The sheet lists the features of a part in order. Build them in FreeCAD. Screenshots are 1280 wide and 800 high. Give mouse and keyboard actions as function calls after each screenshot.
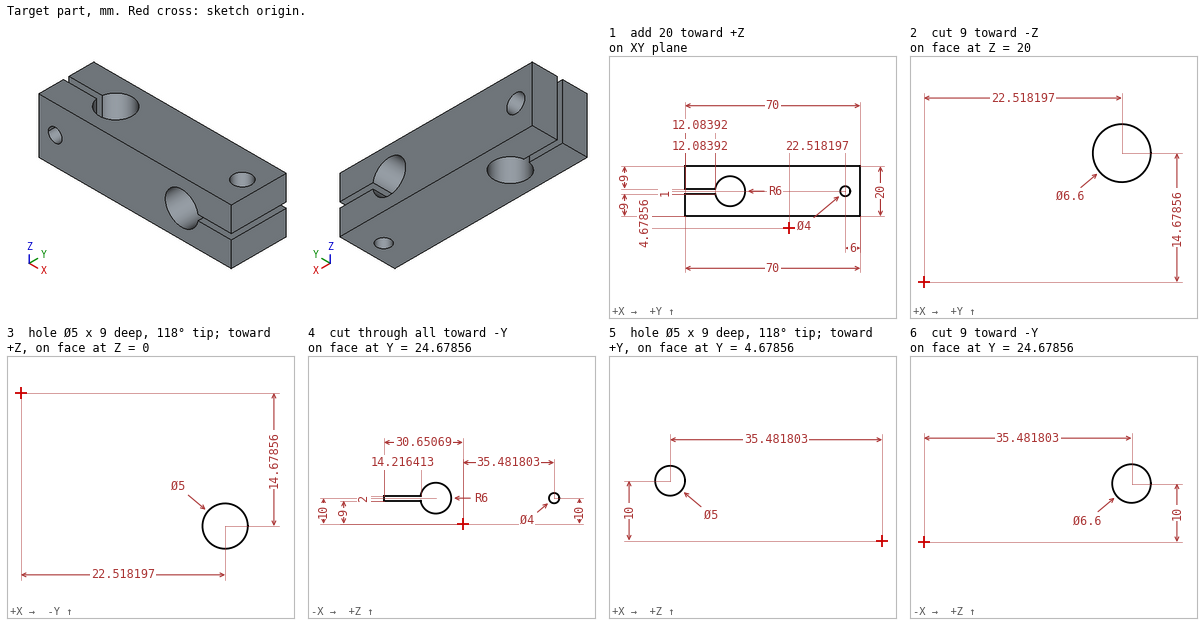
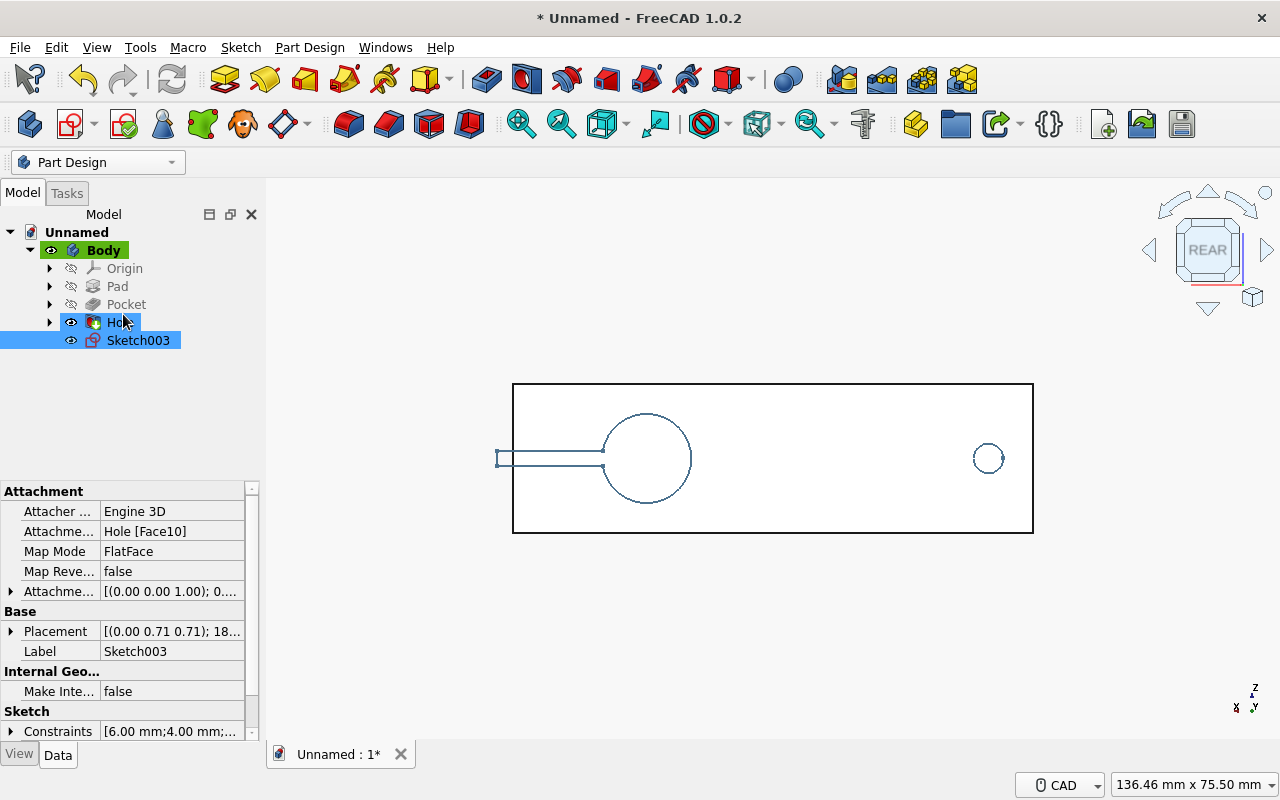
click(488, 80)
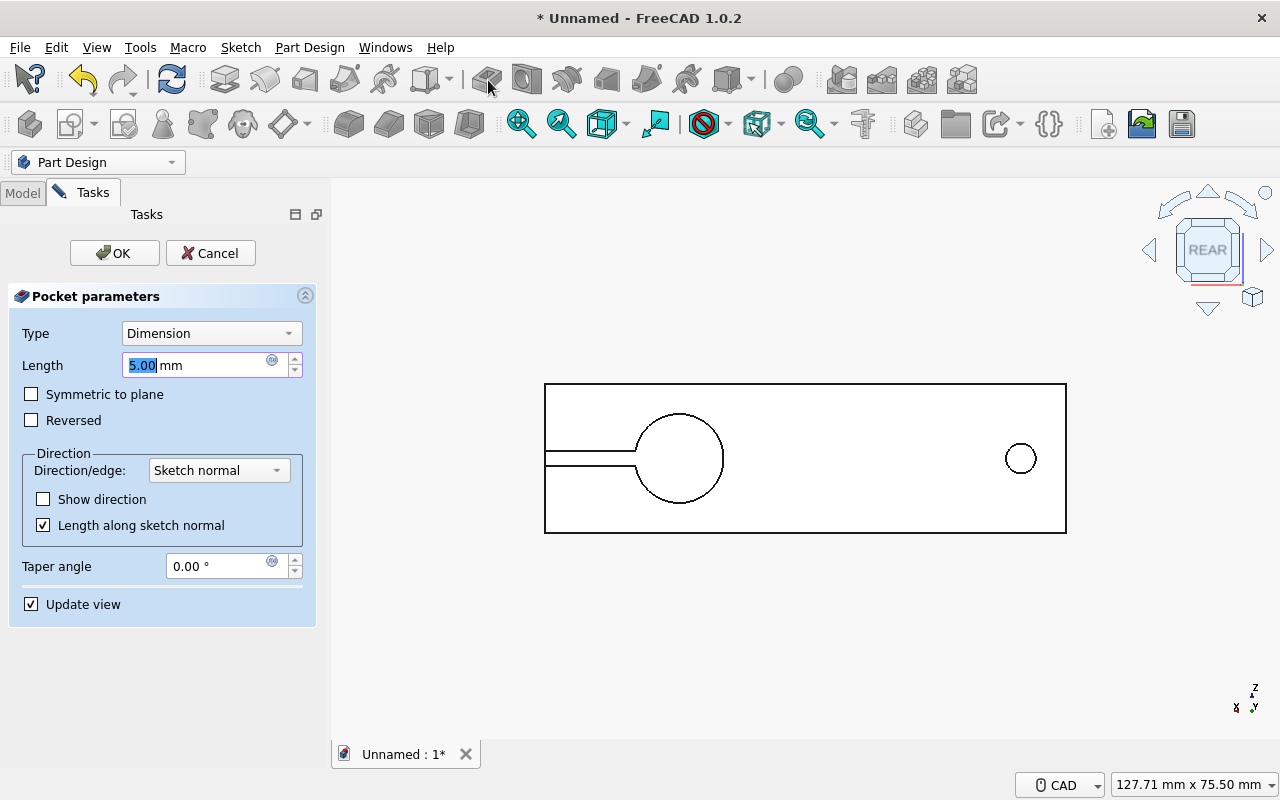
click(212, 334)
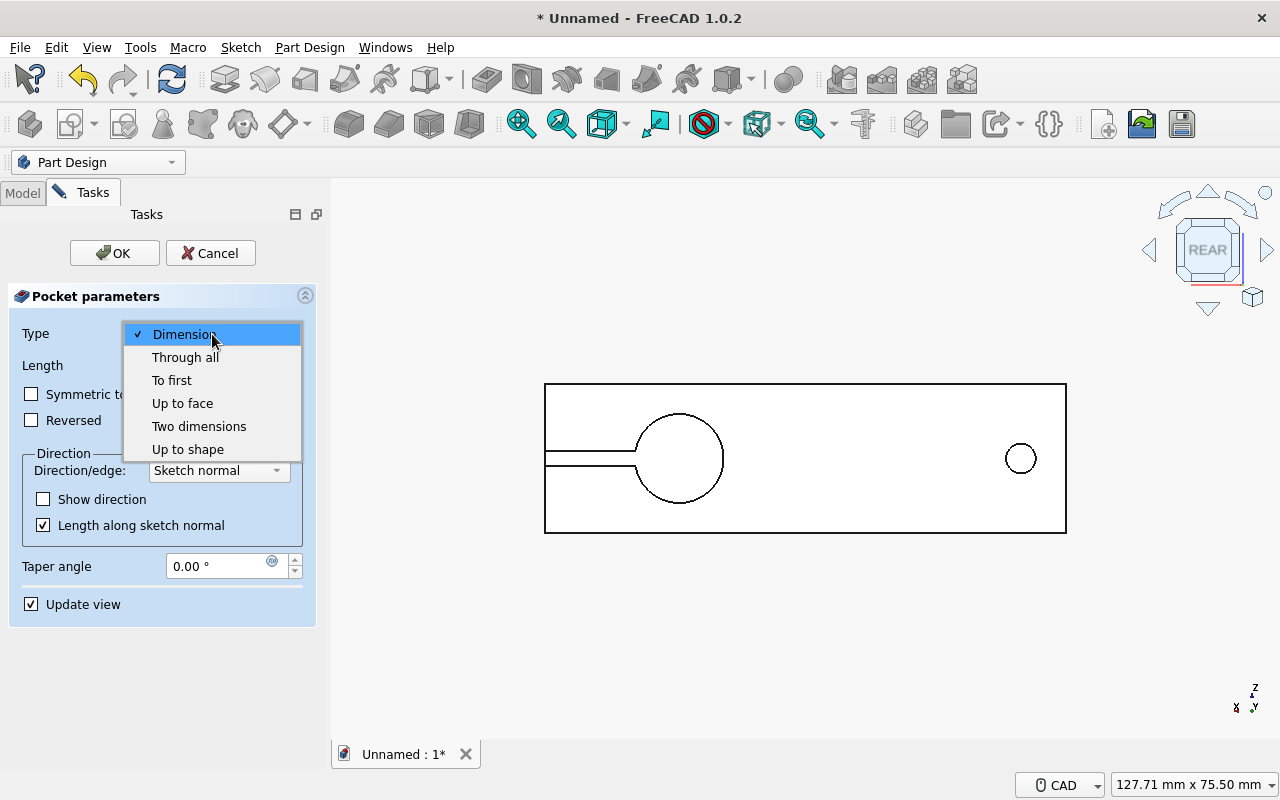
click(212, 358)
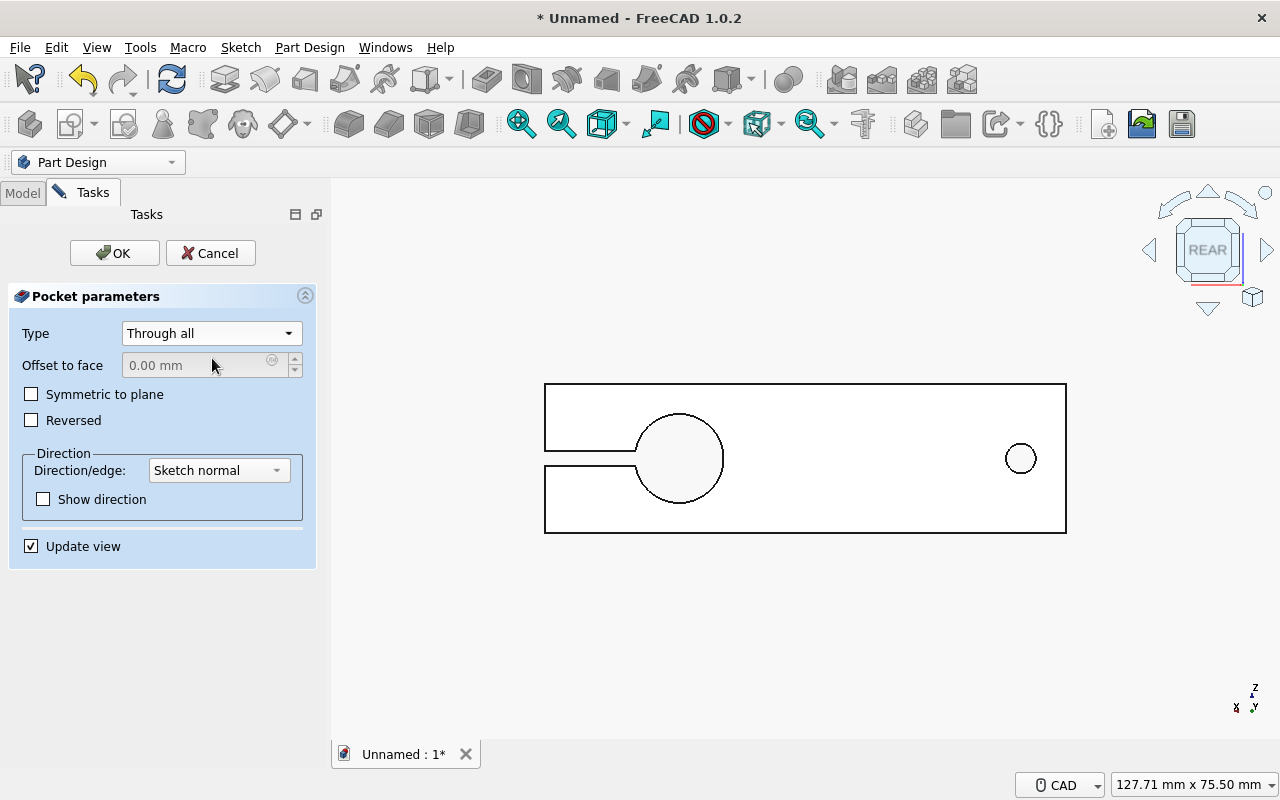
click(115, 253)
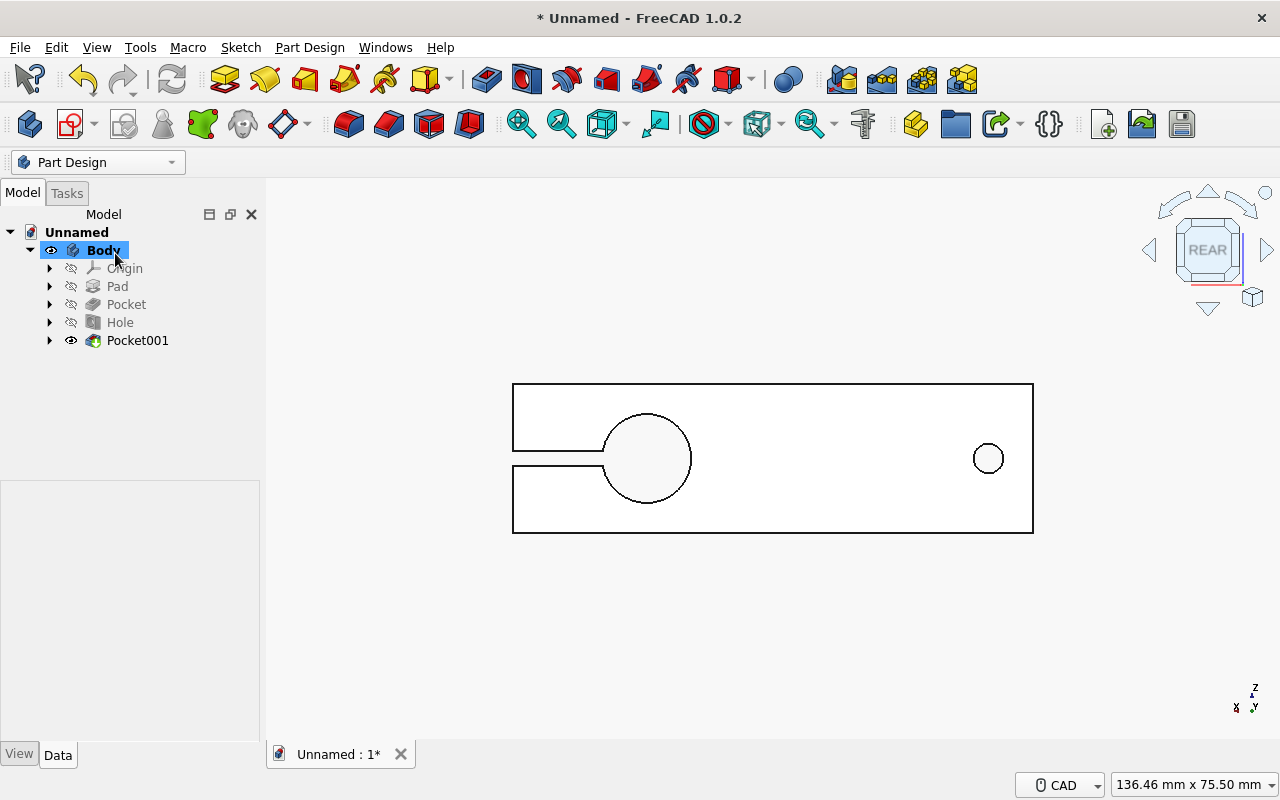
key(0)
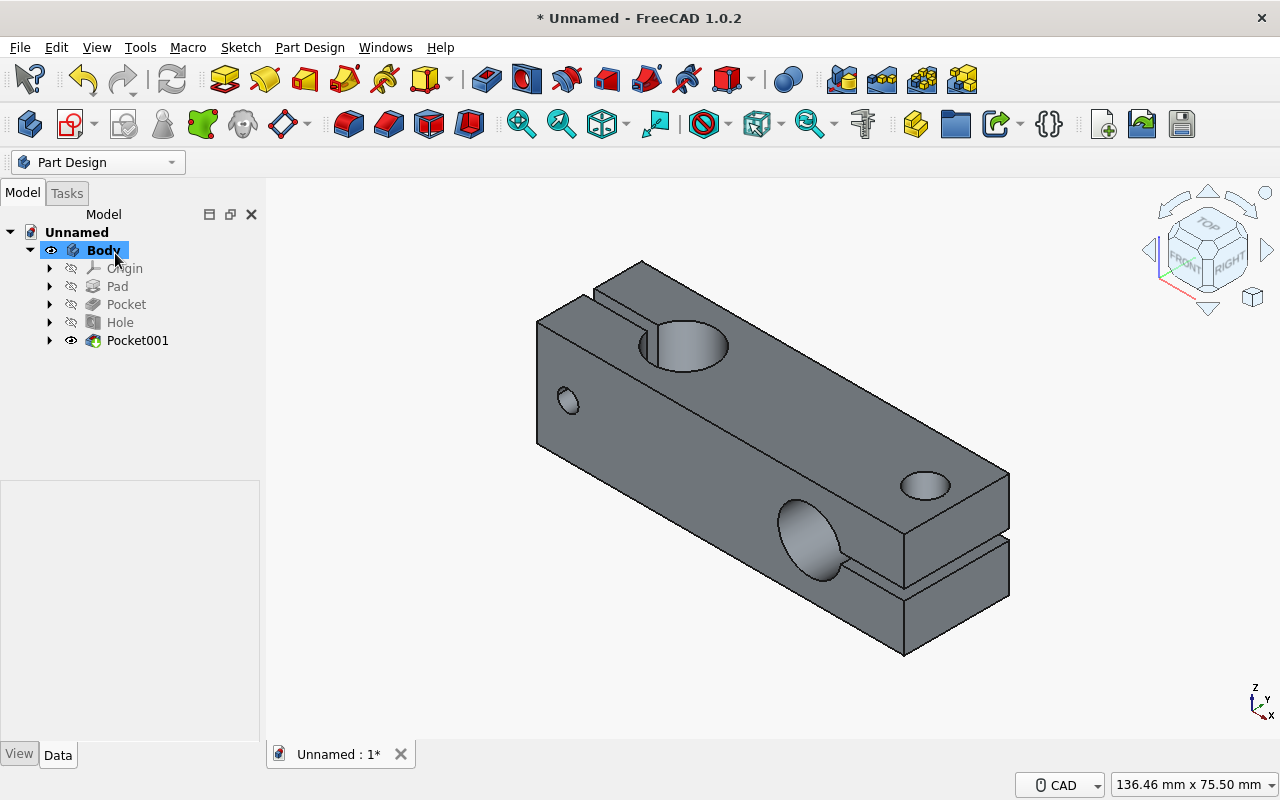
click(720, 488)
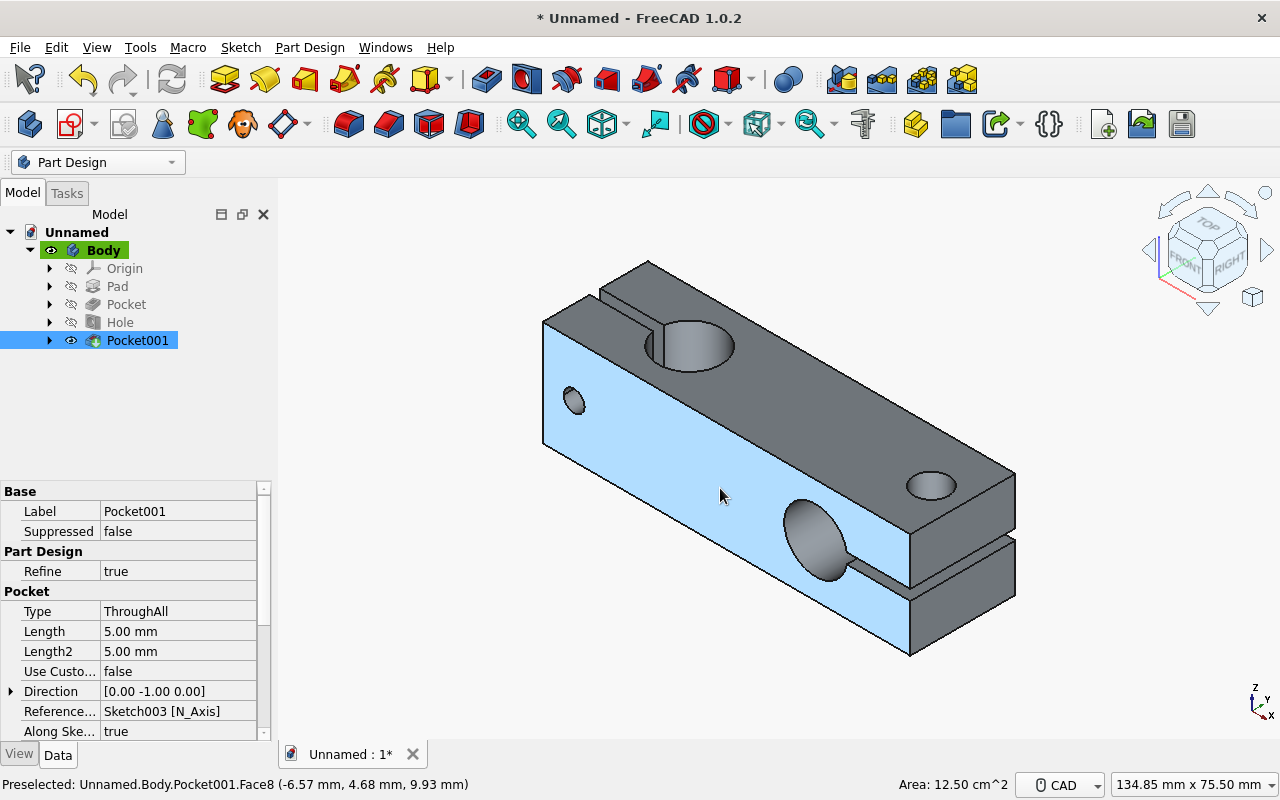
click(70, 124)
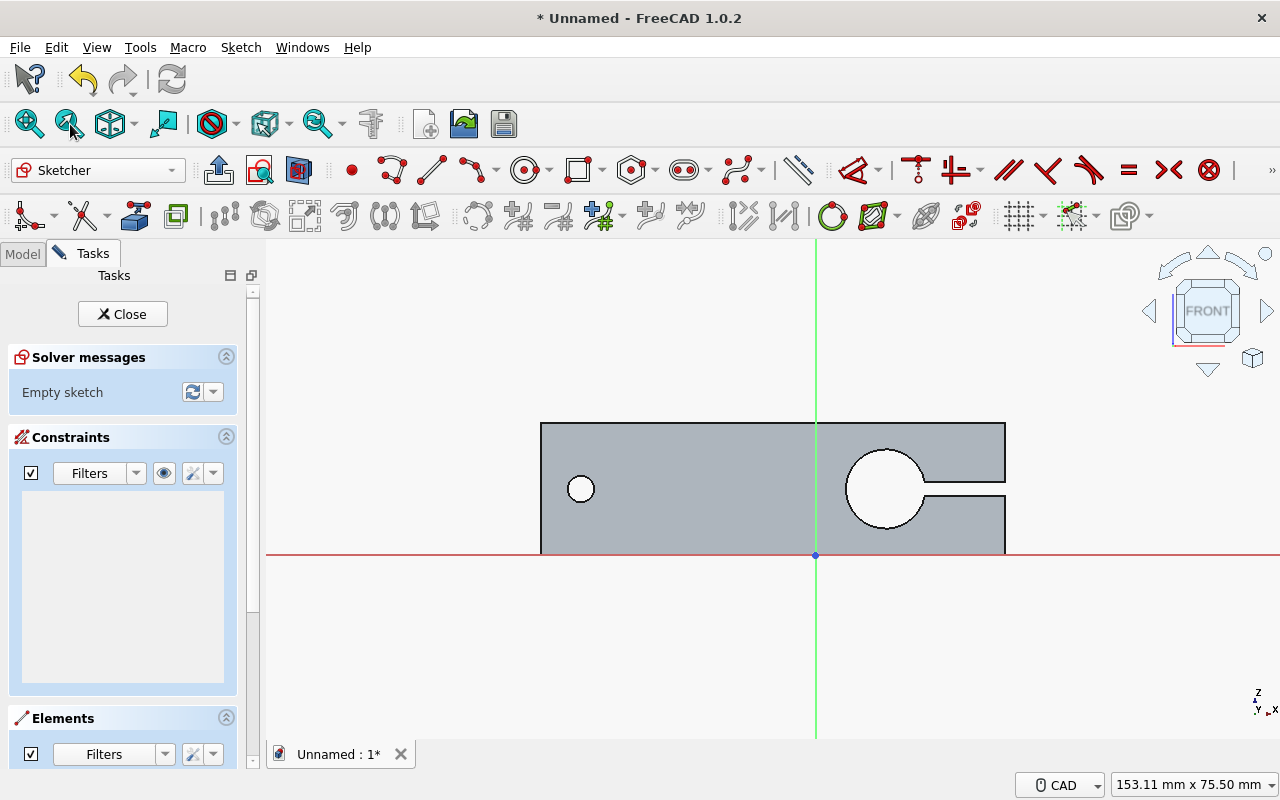
scroll(566, 489, up, 11)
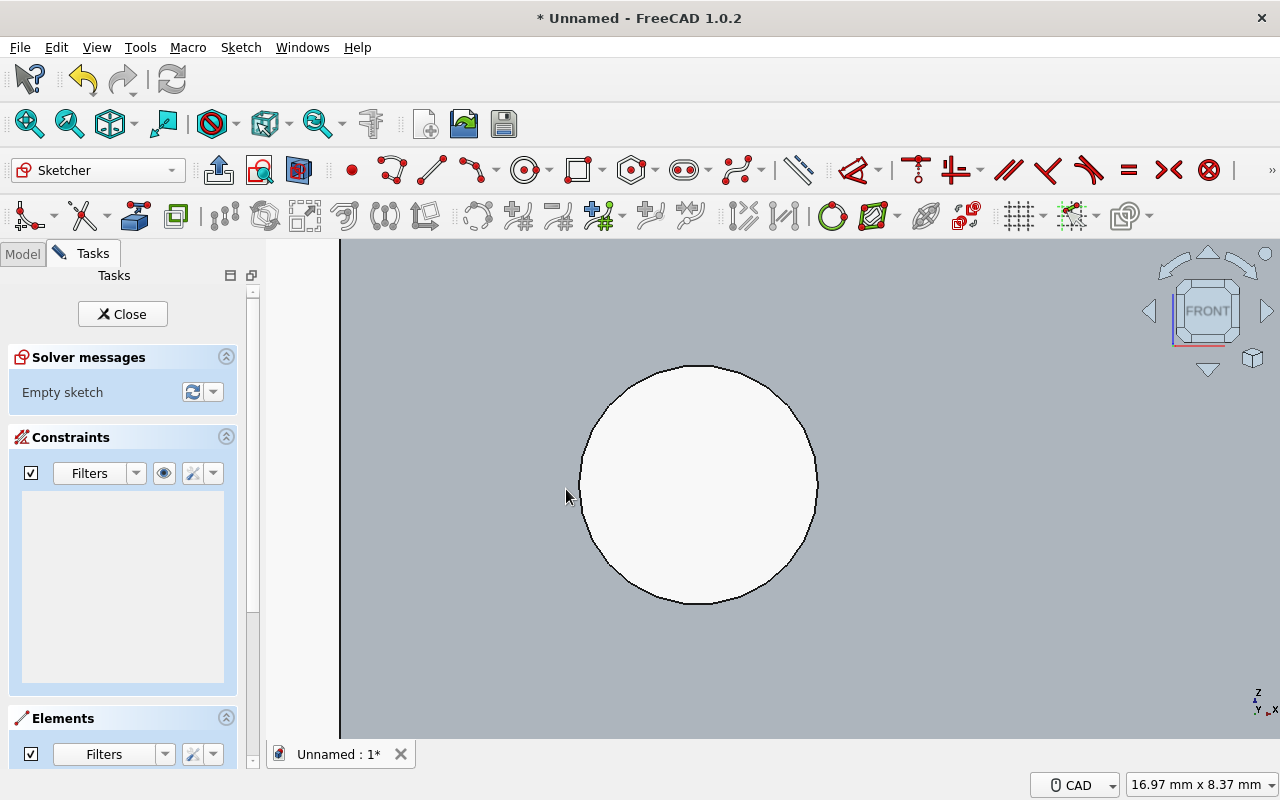
key(g)
key(c)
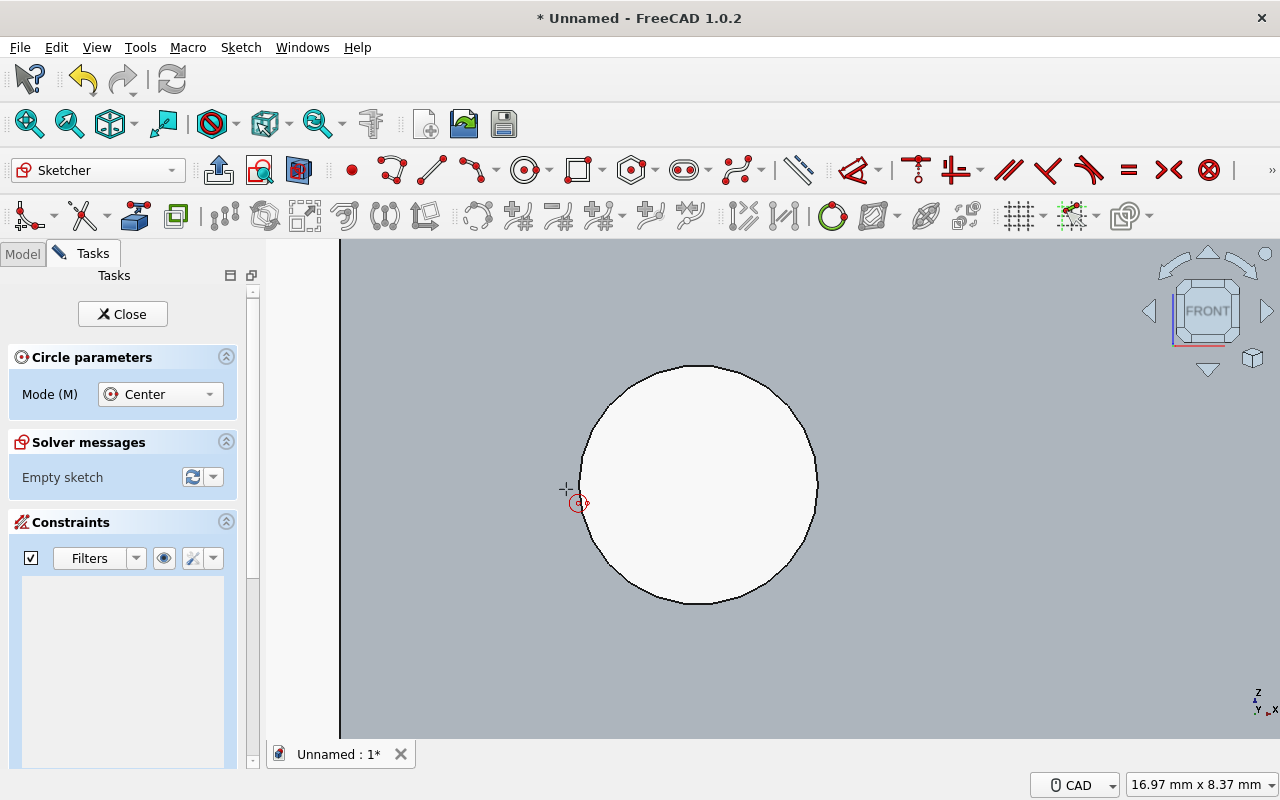
click(698, 485)
click(804, 379)
key(Escape)